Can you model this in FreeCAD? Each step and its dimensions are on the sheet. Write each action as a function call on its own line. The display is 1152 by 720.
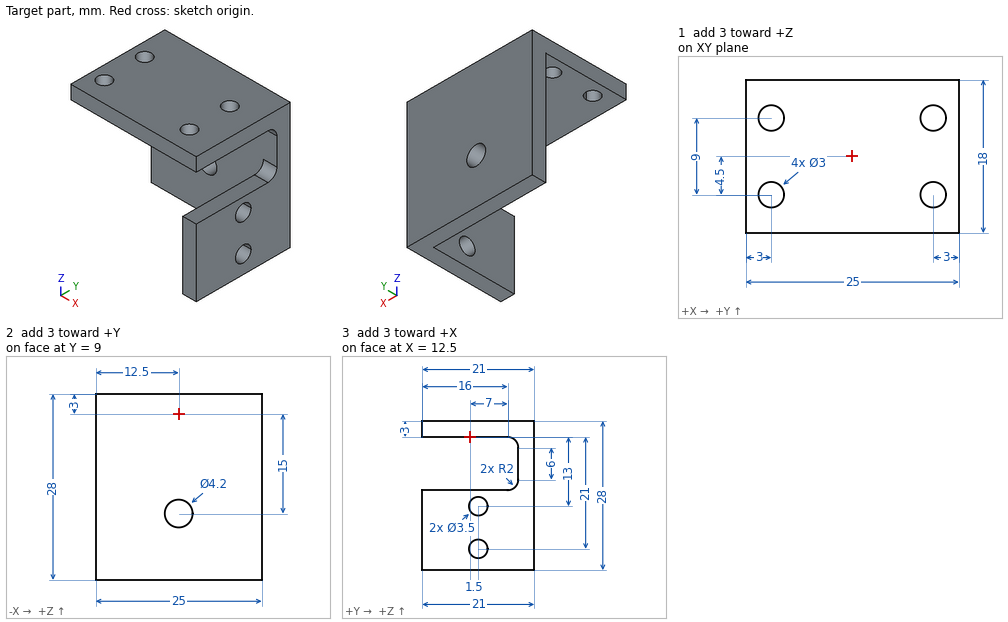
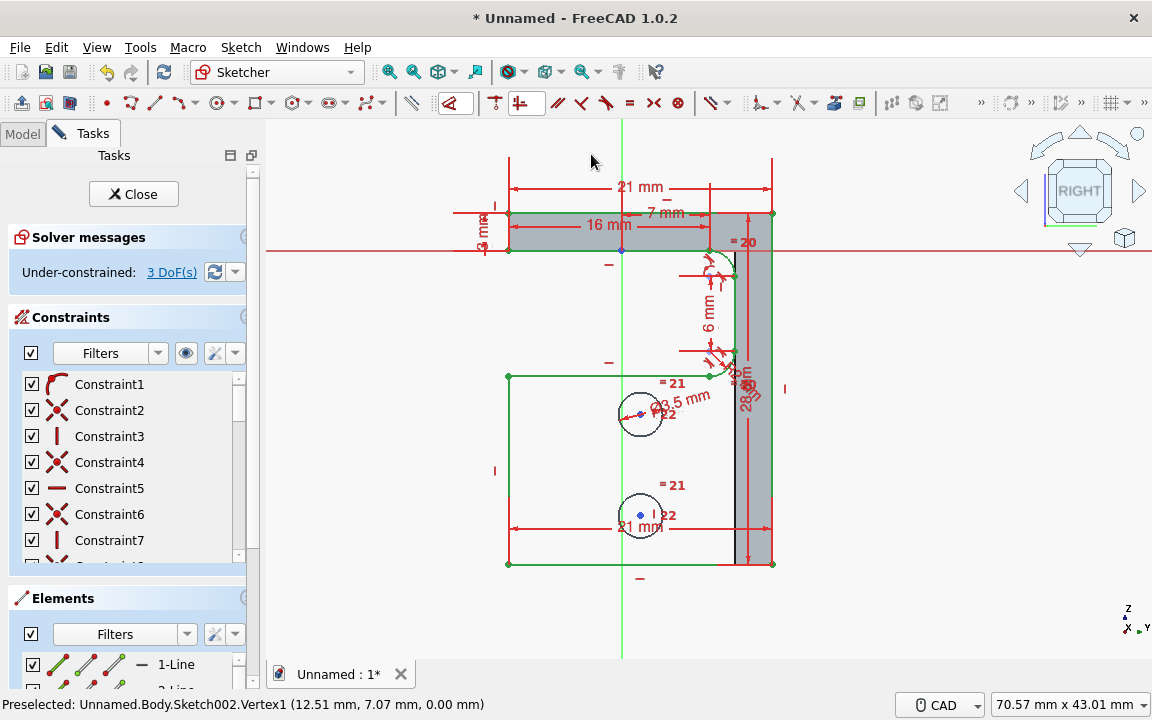
click(641, 415)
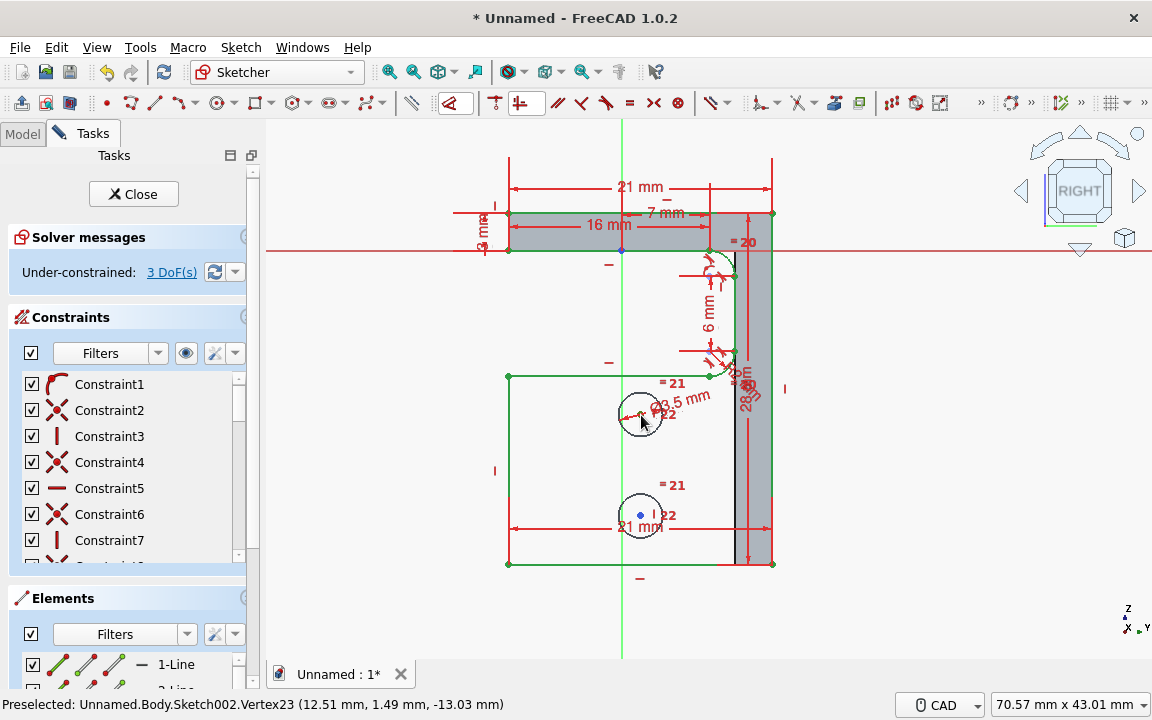
key(i)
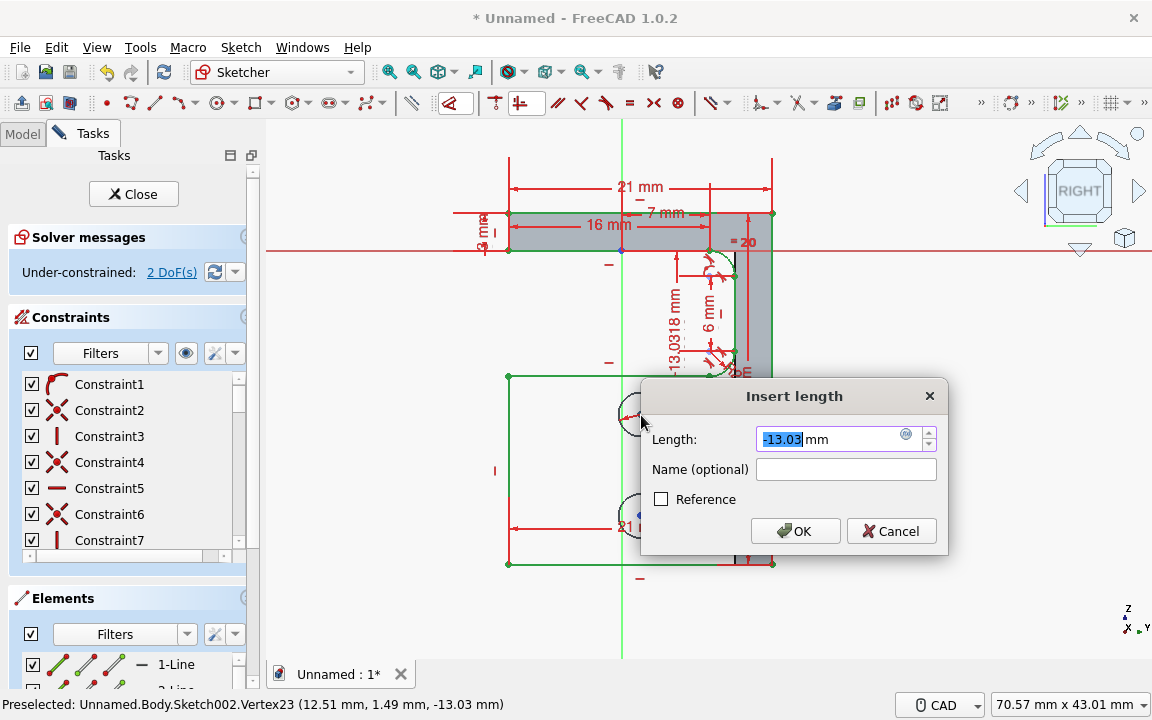
text(-13)
key(Return)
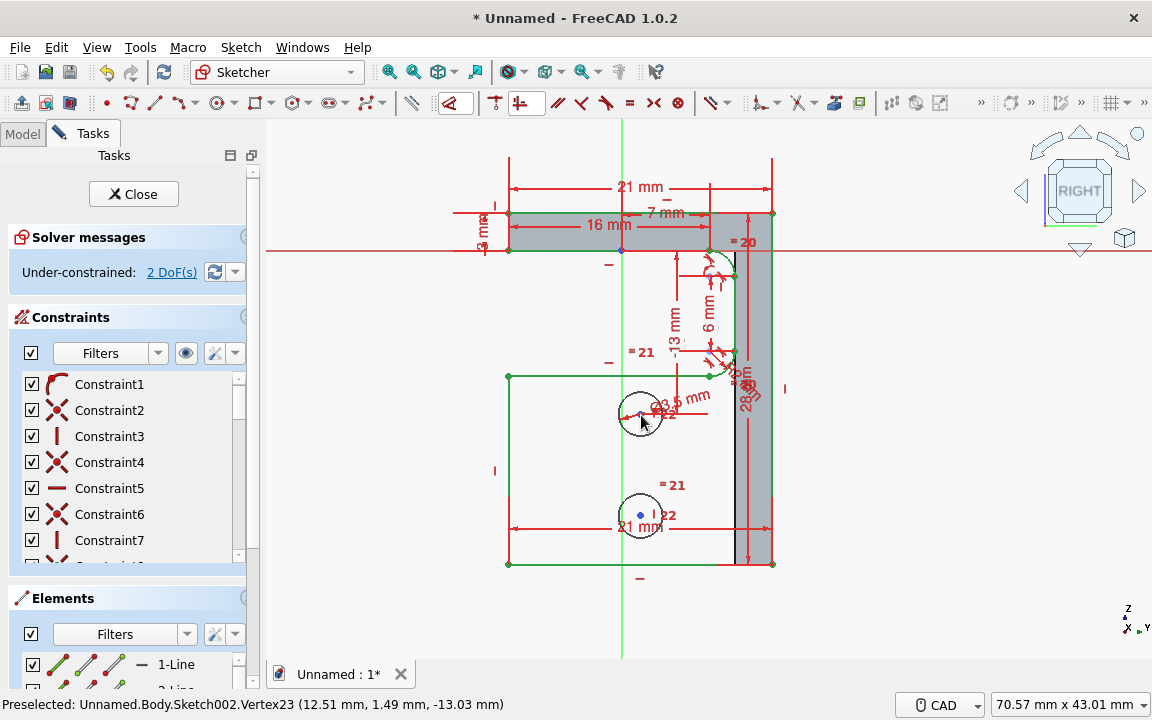
click(641, 516)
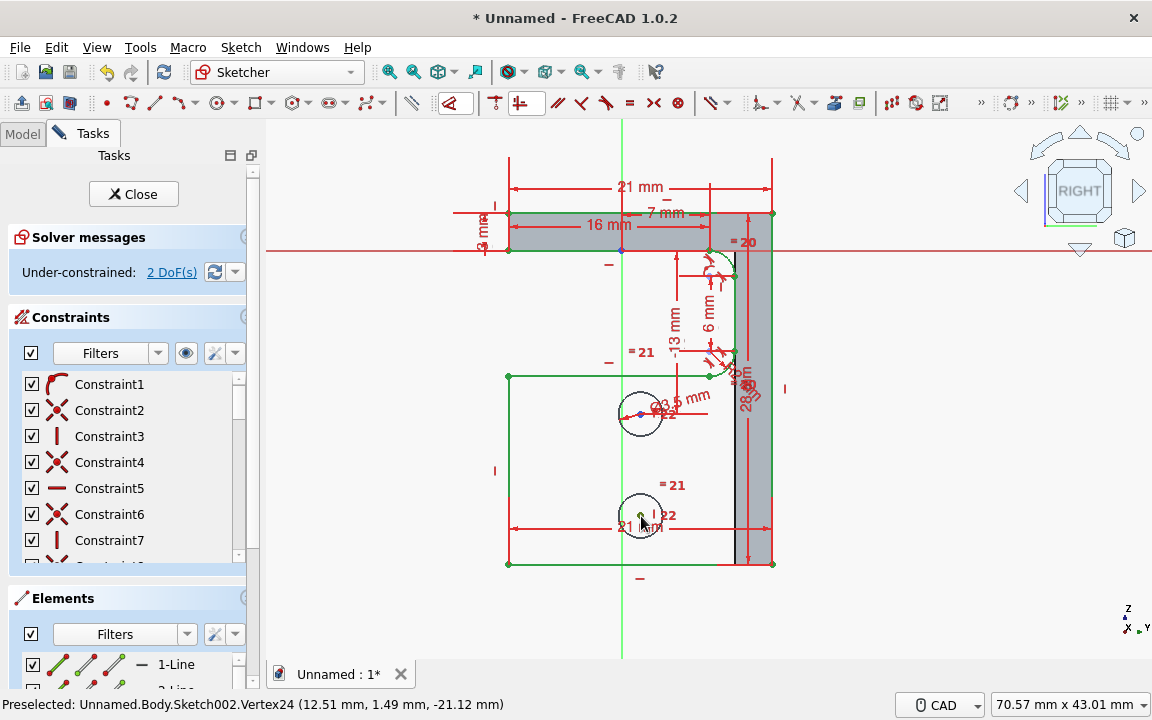
key(i)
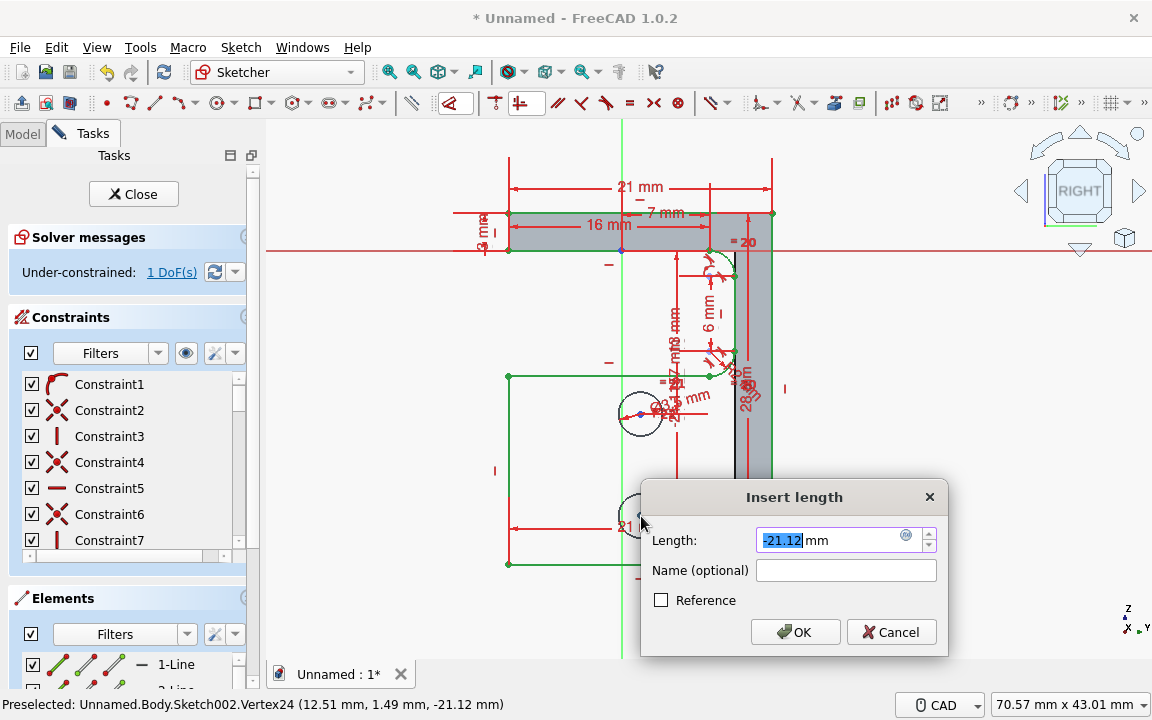
text(-21)
key(Return)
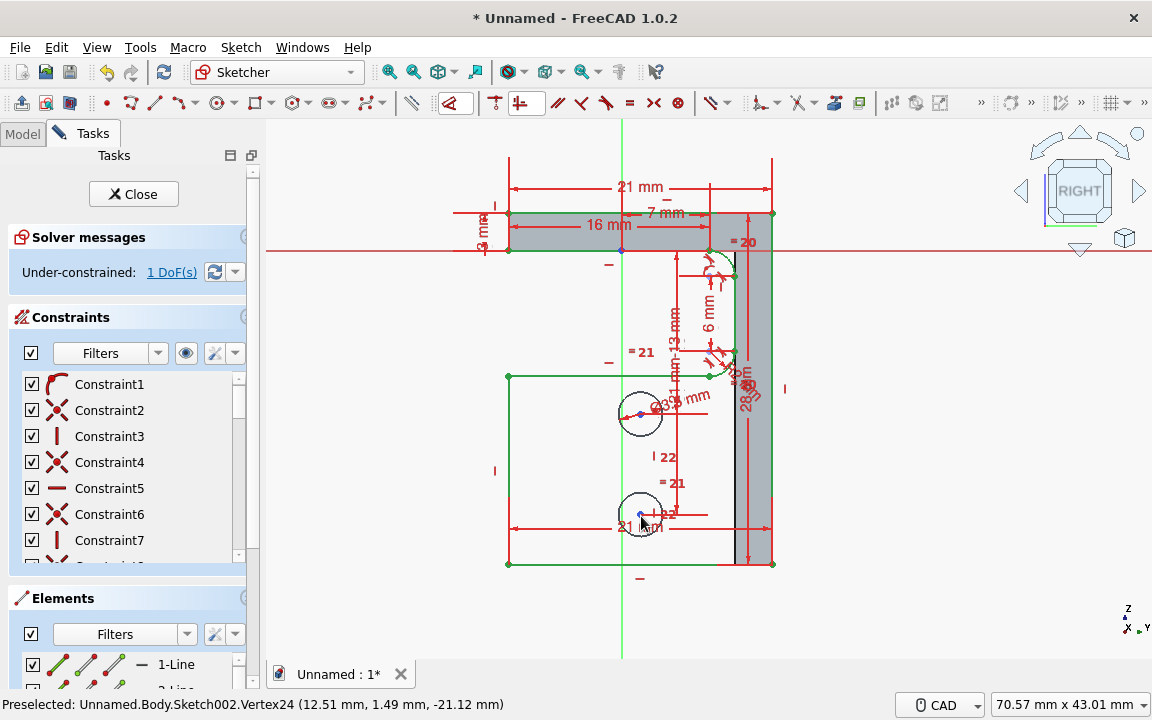
scroll(641, 414, up, 4)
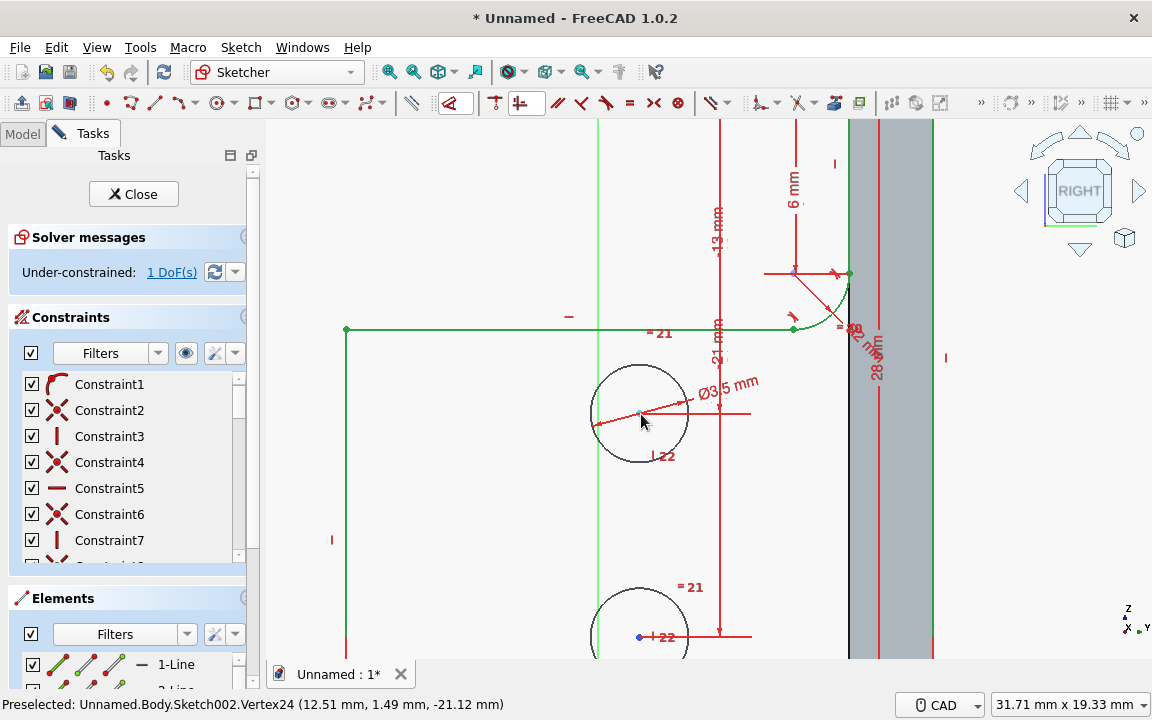
click(640, 414)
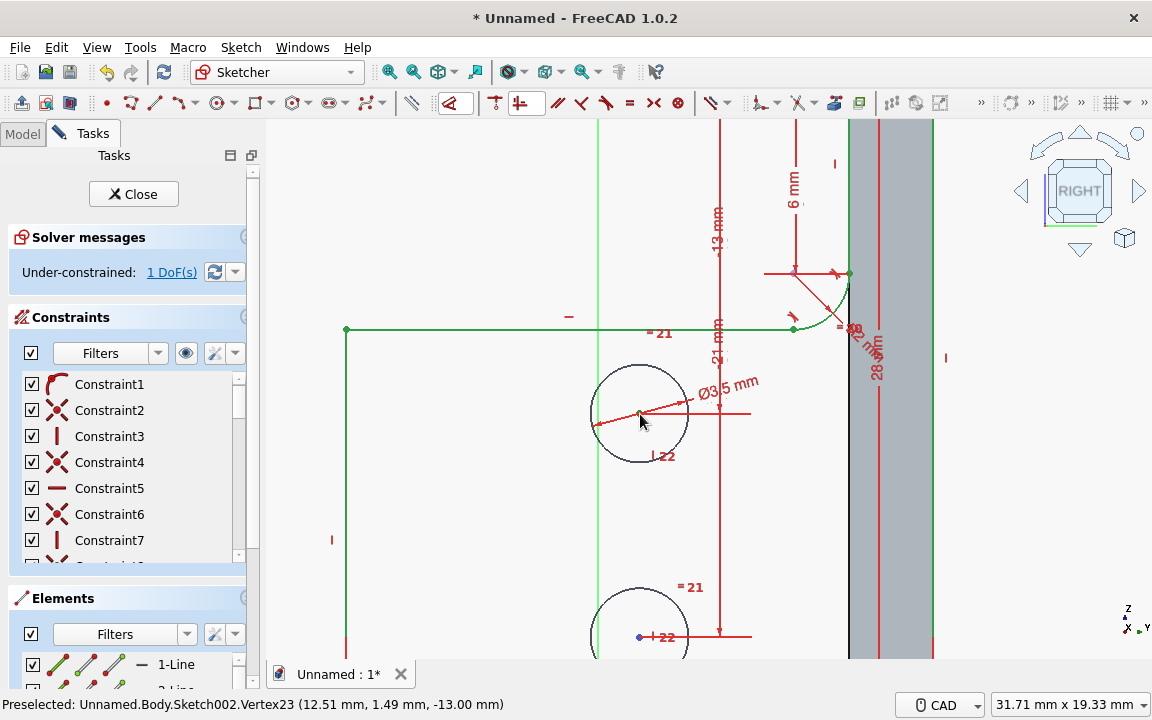
key(l)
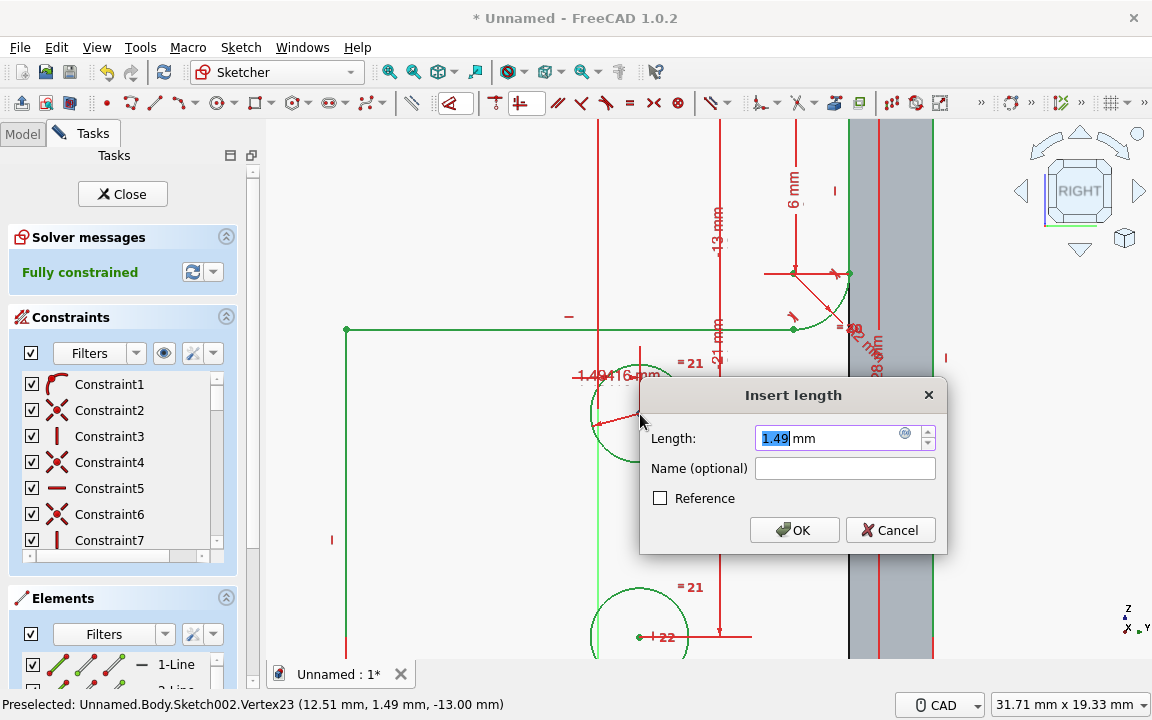
text(1.5)
key(Return)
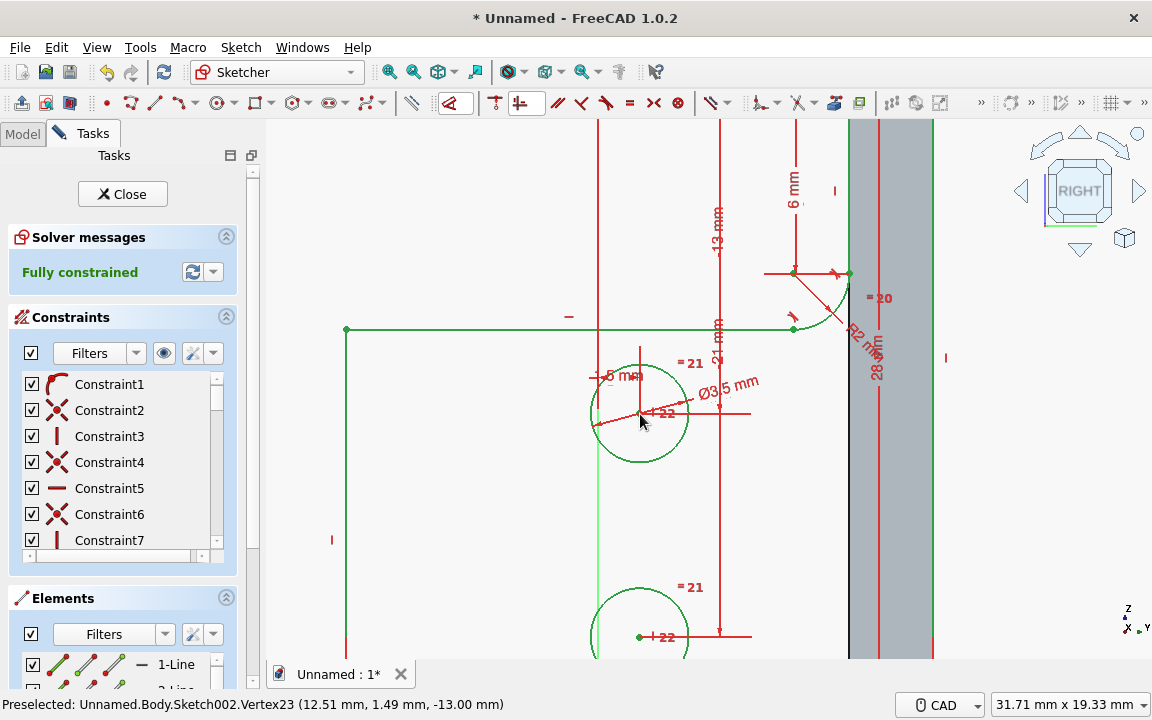
click(123, 194)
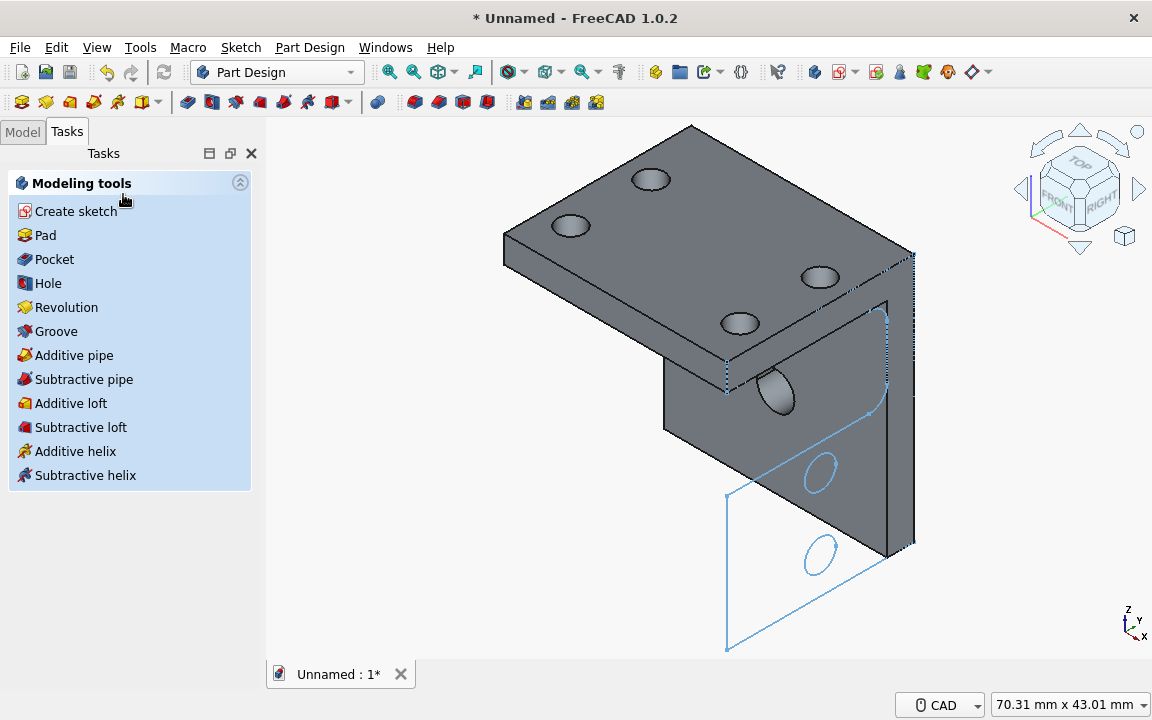
click(22, 102)